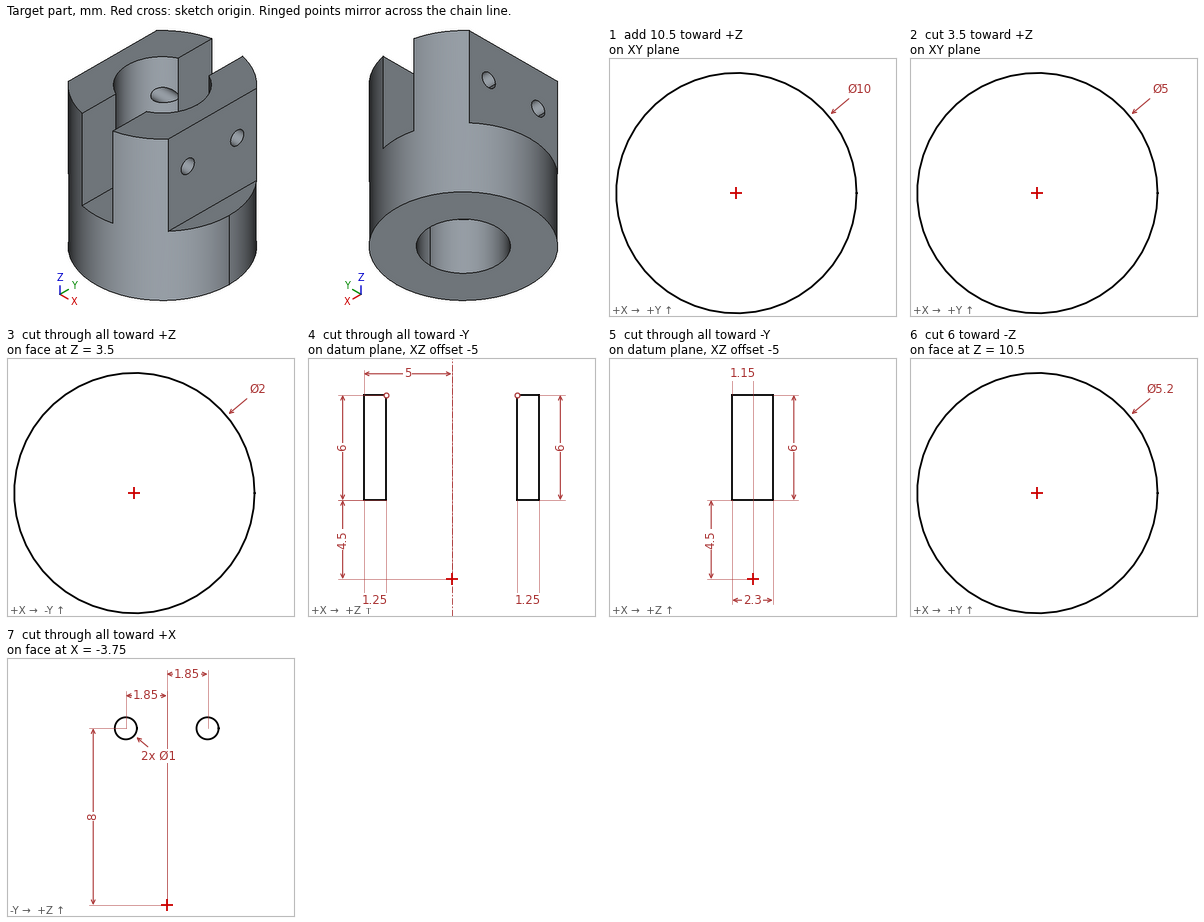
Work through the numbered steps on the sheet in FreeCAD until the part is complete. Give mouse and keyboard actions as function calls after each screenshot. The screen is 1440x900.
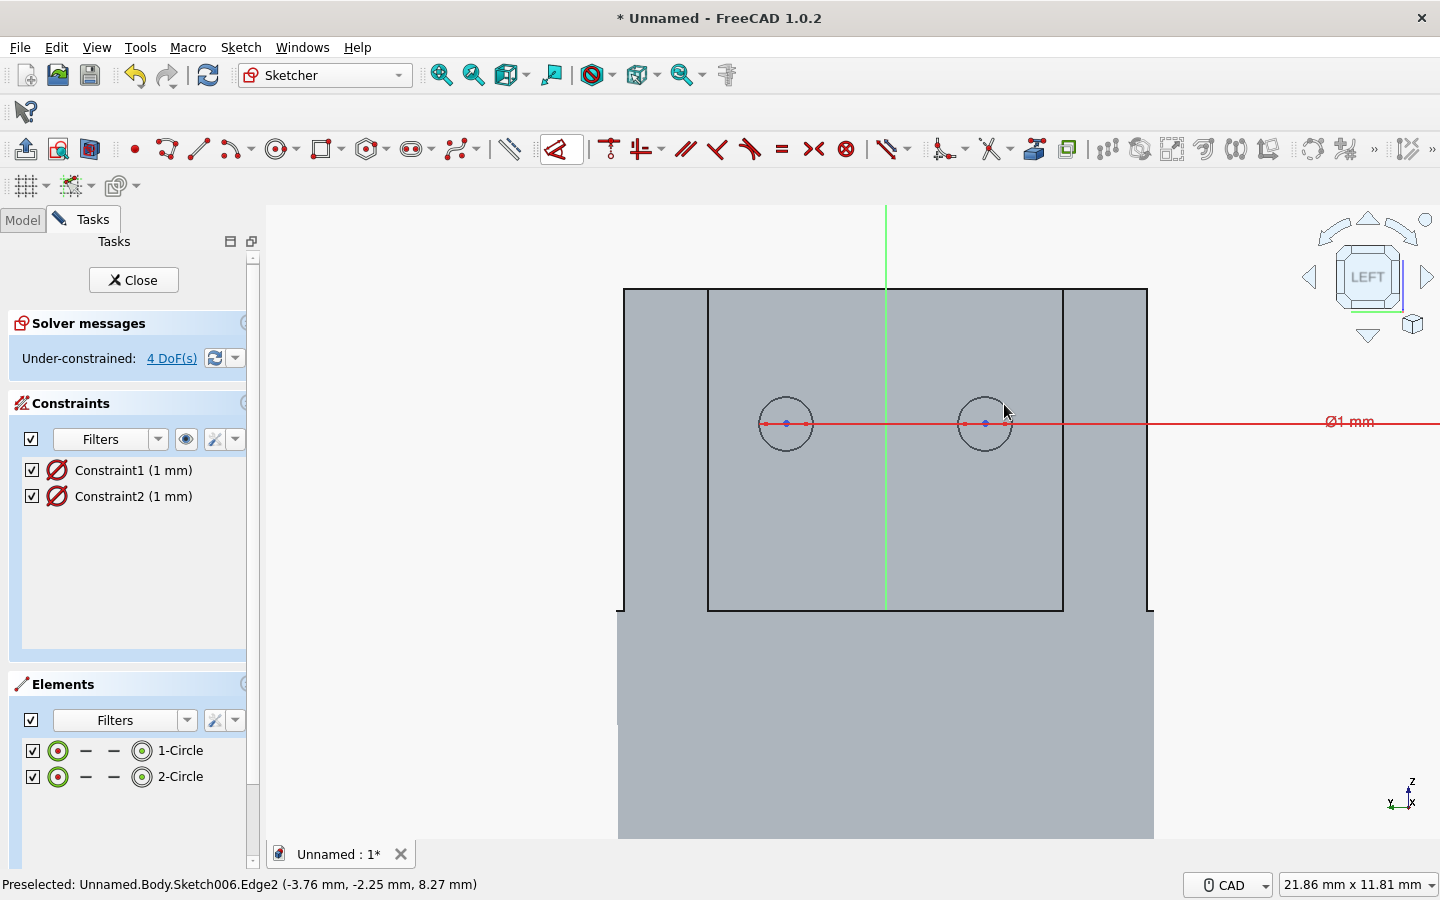
click(786, 424)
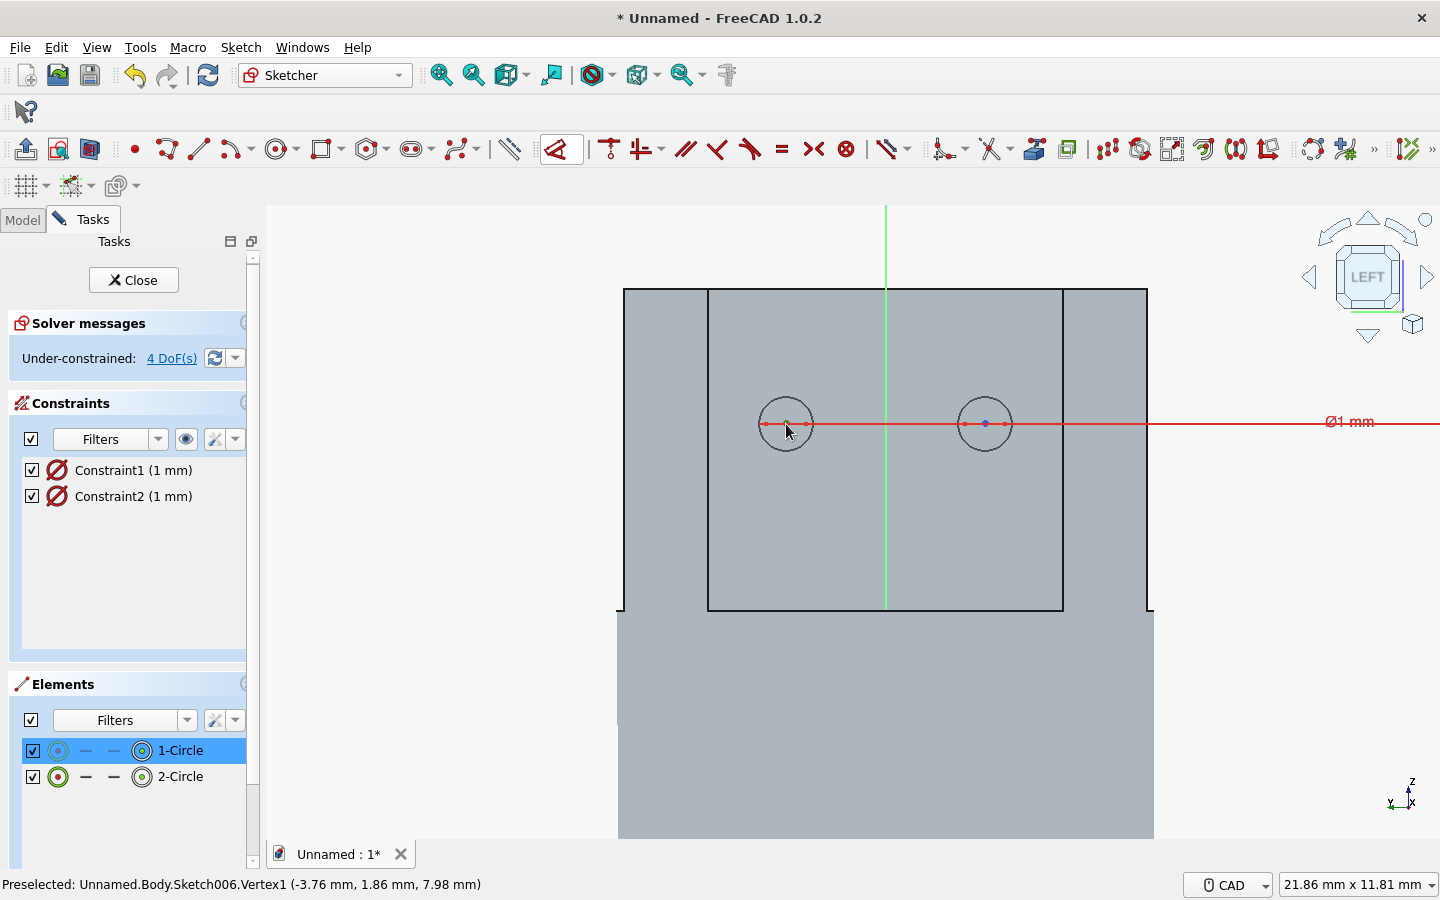
click(985, 424)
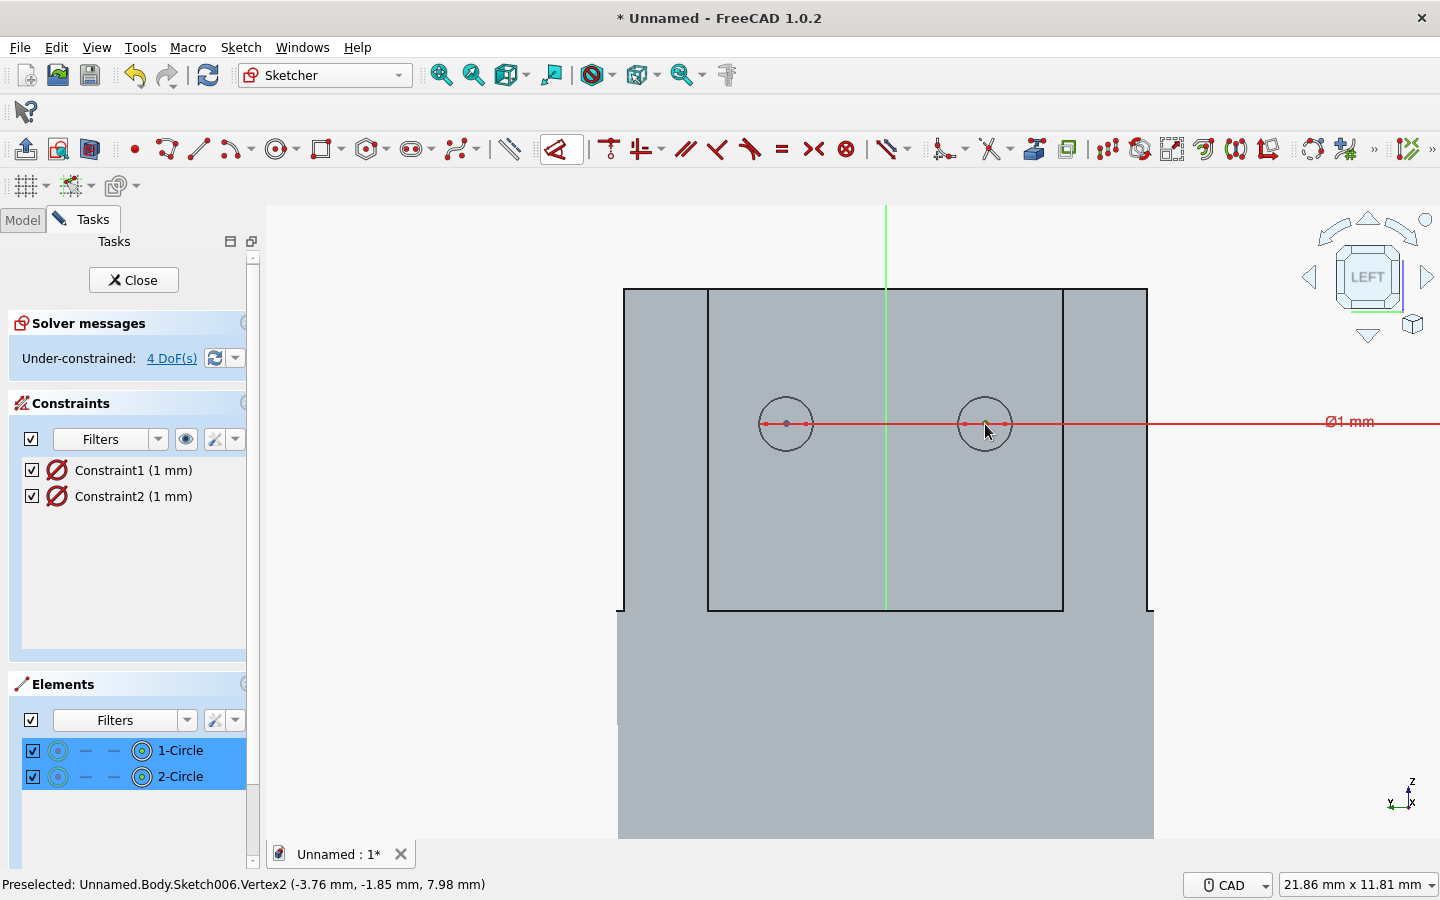
click(664, 150)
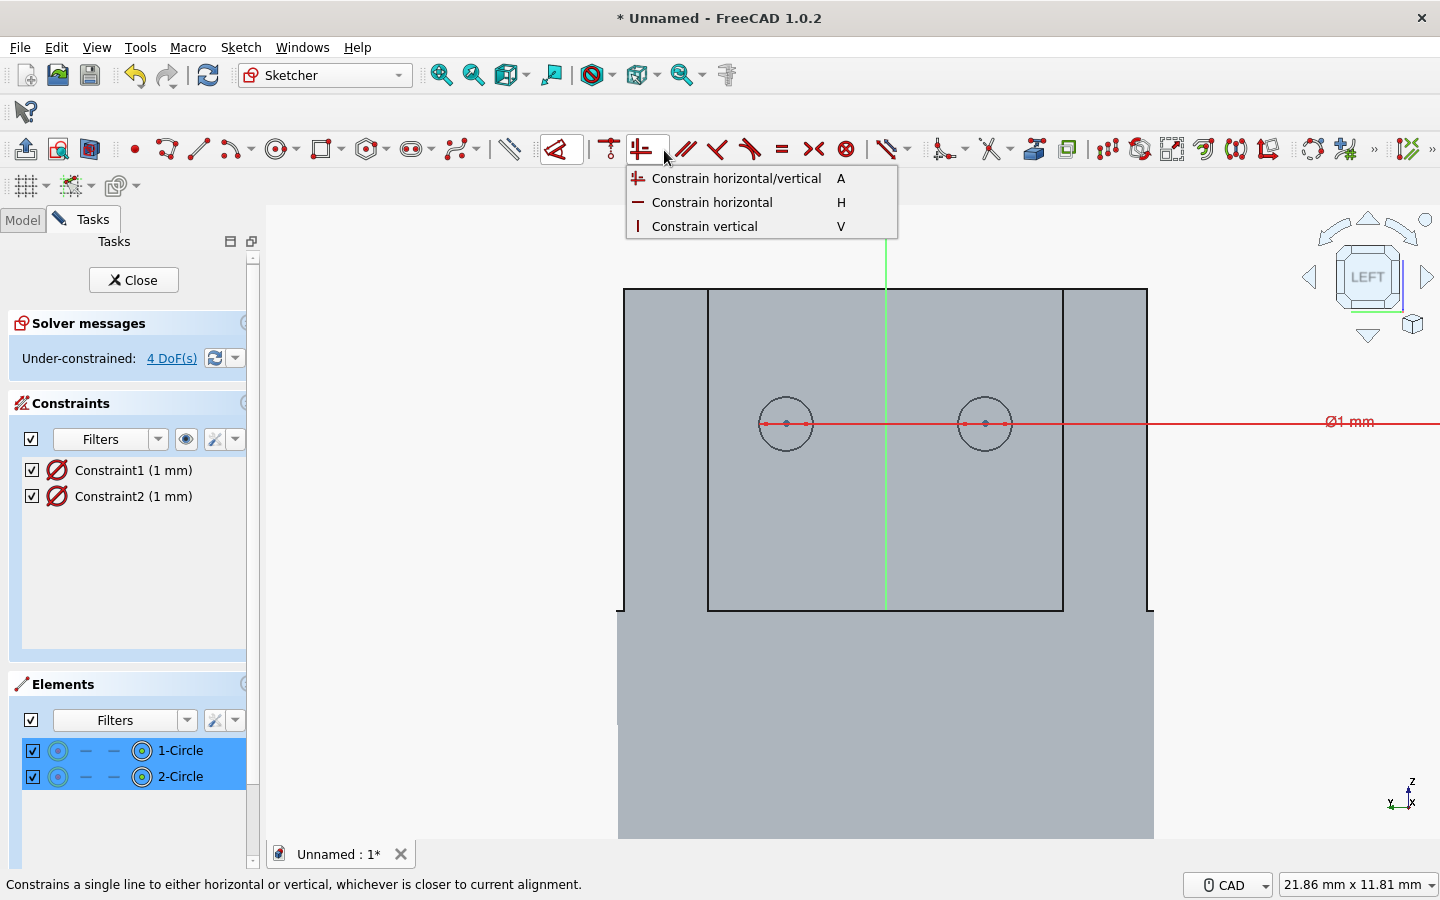
click(762, 202)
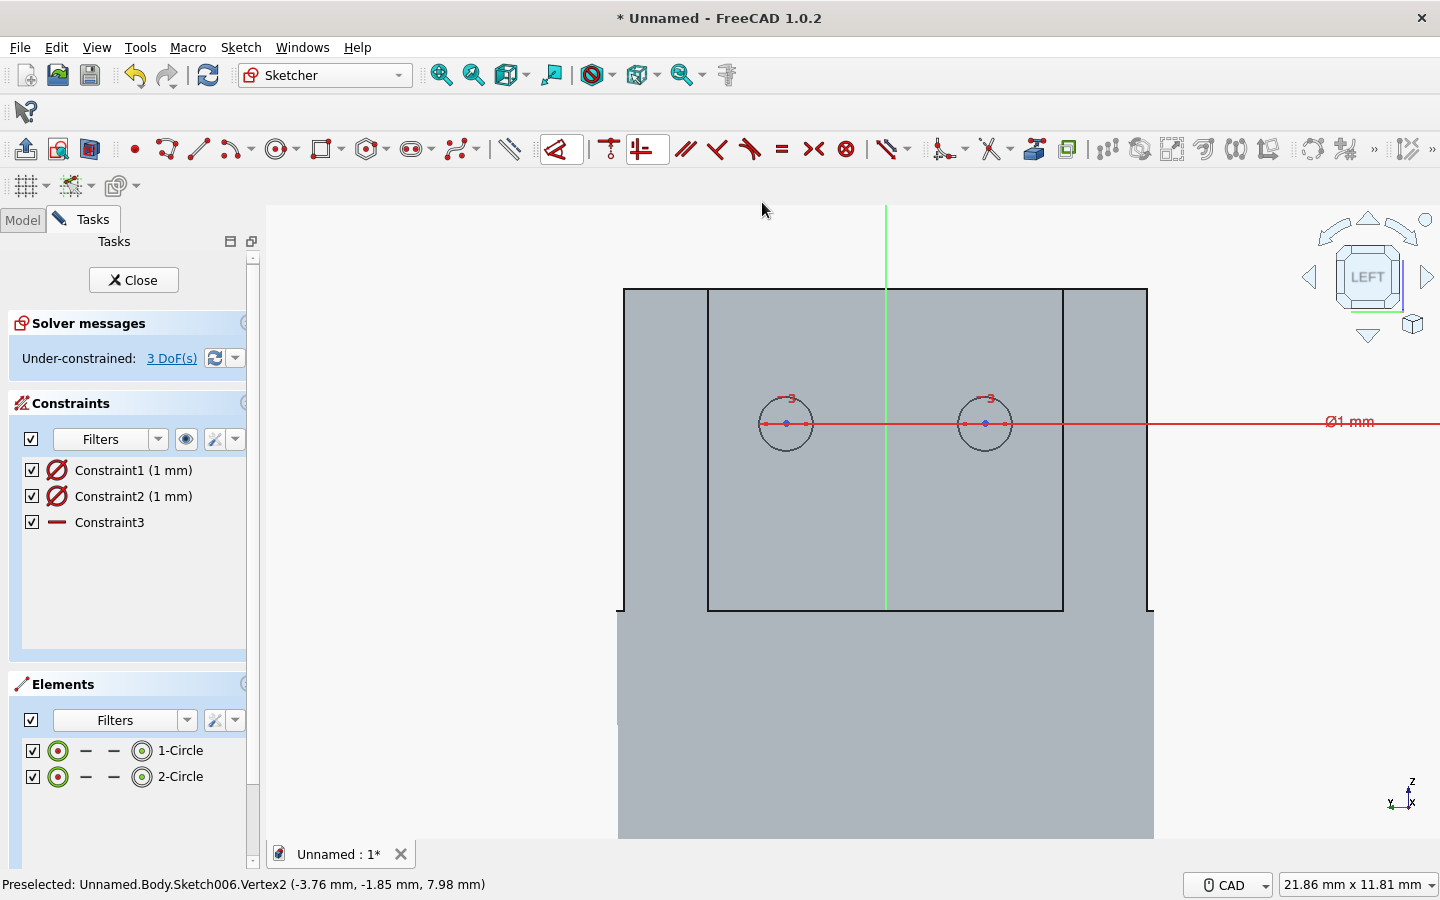
click(786, 424)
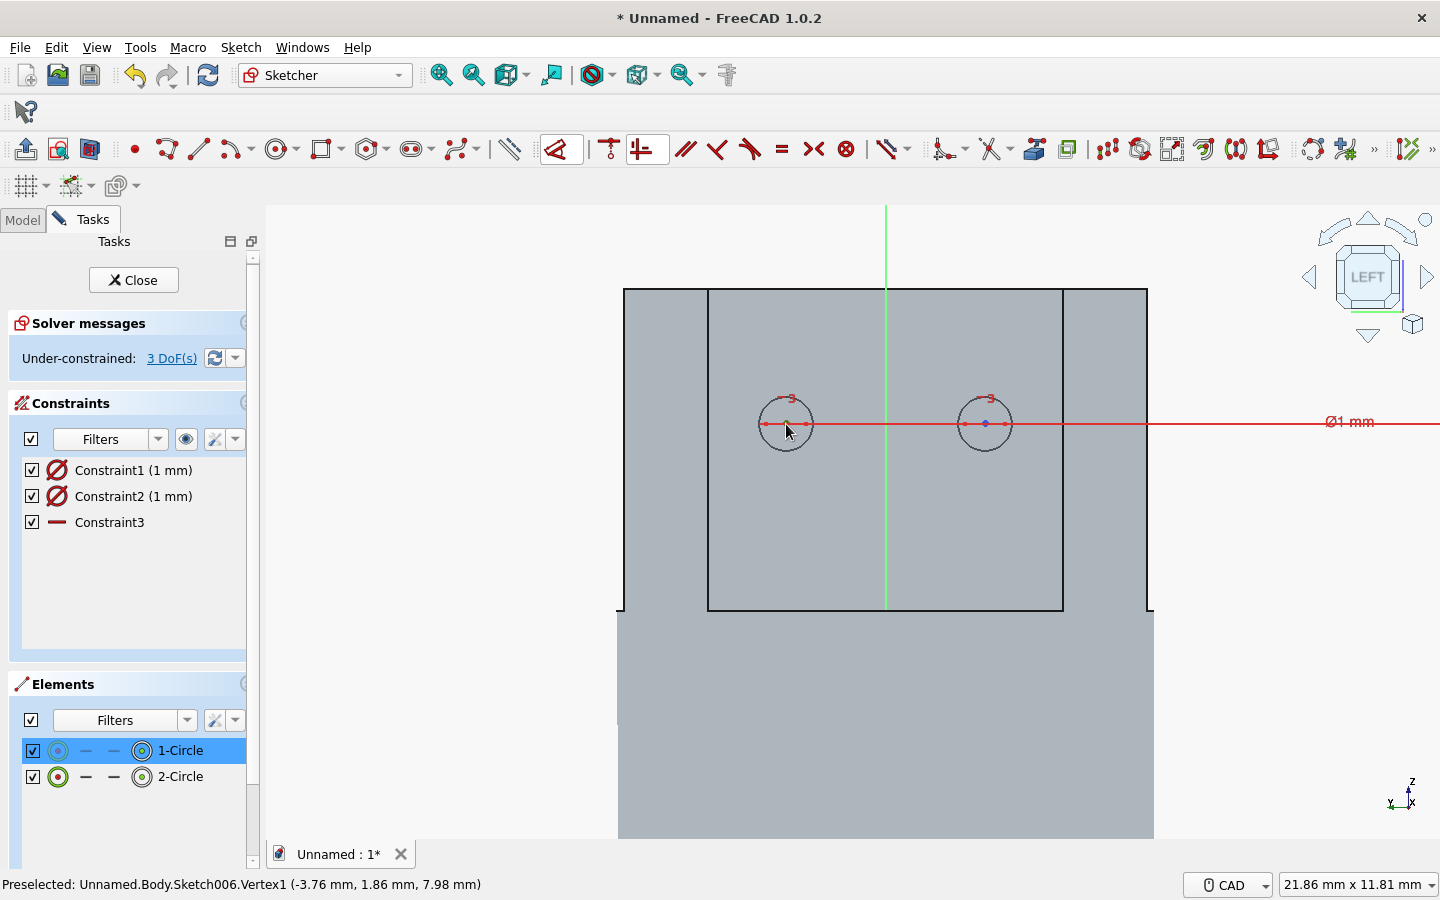
key(i)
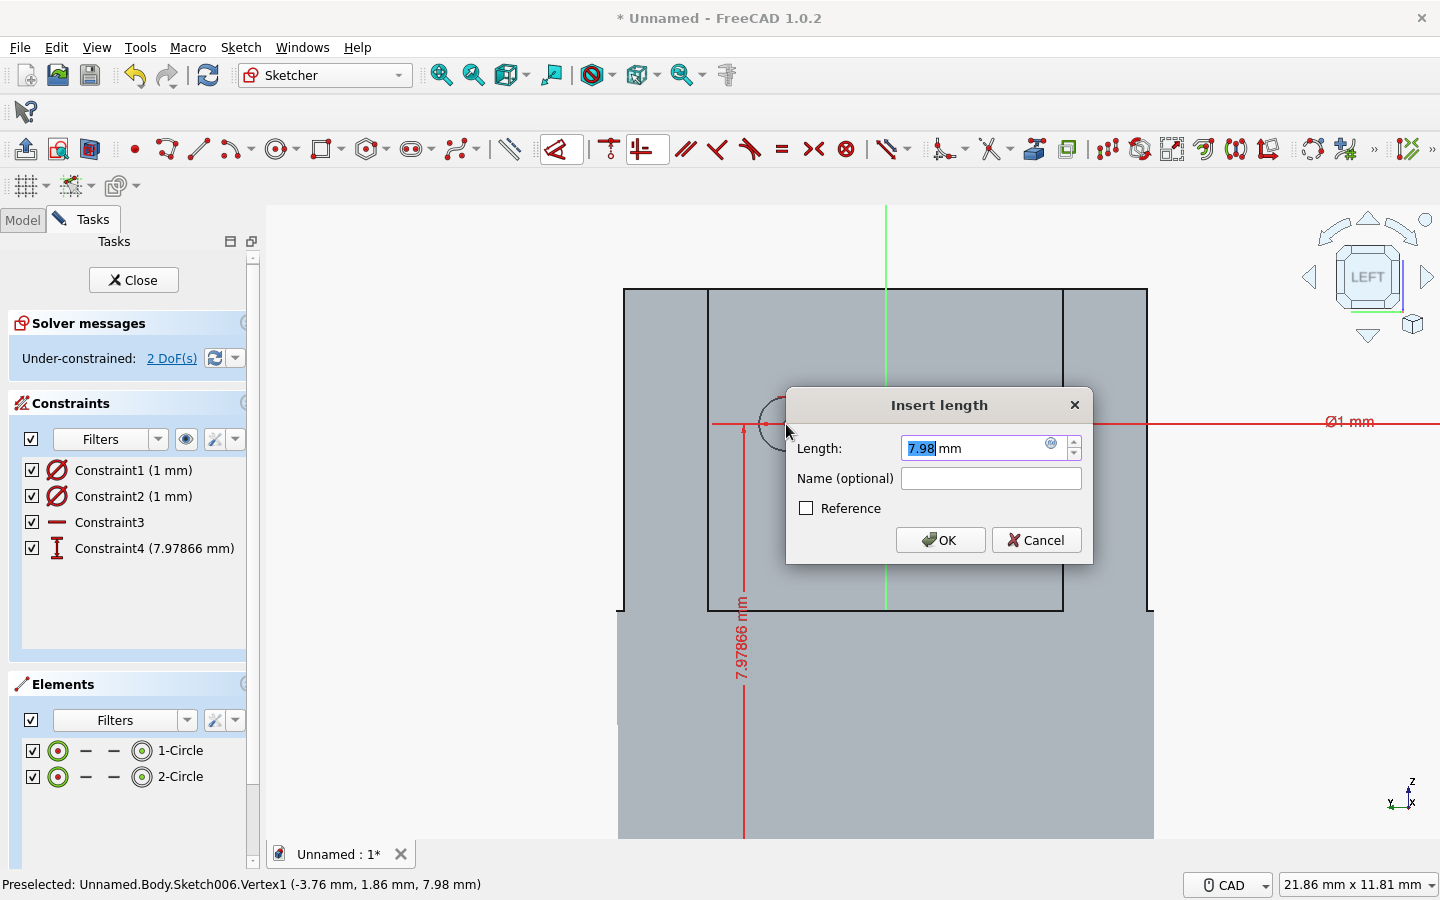
text(8)
key(Return)